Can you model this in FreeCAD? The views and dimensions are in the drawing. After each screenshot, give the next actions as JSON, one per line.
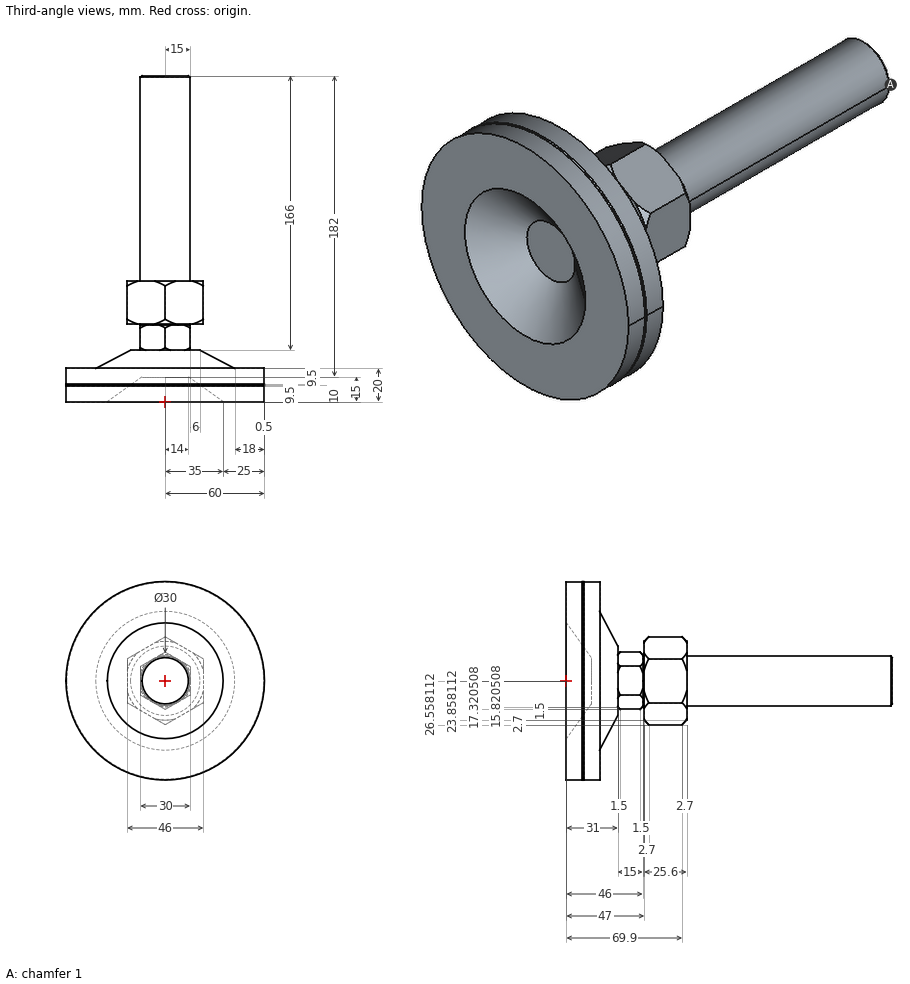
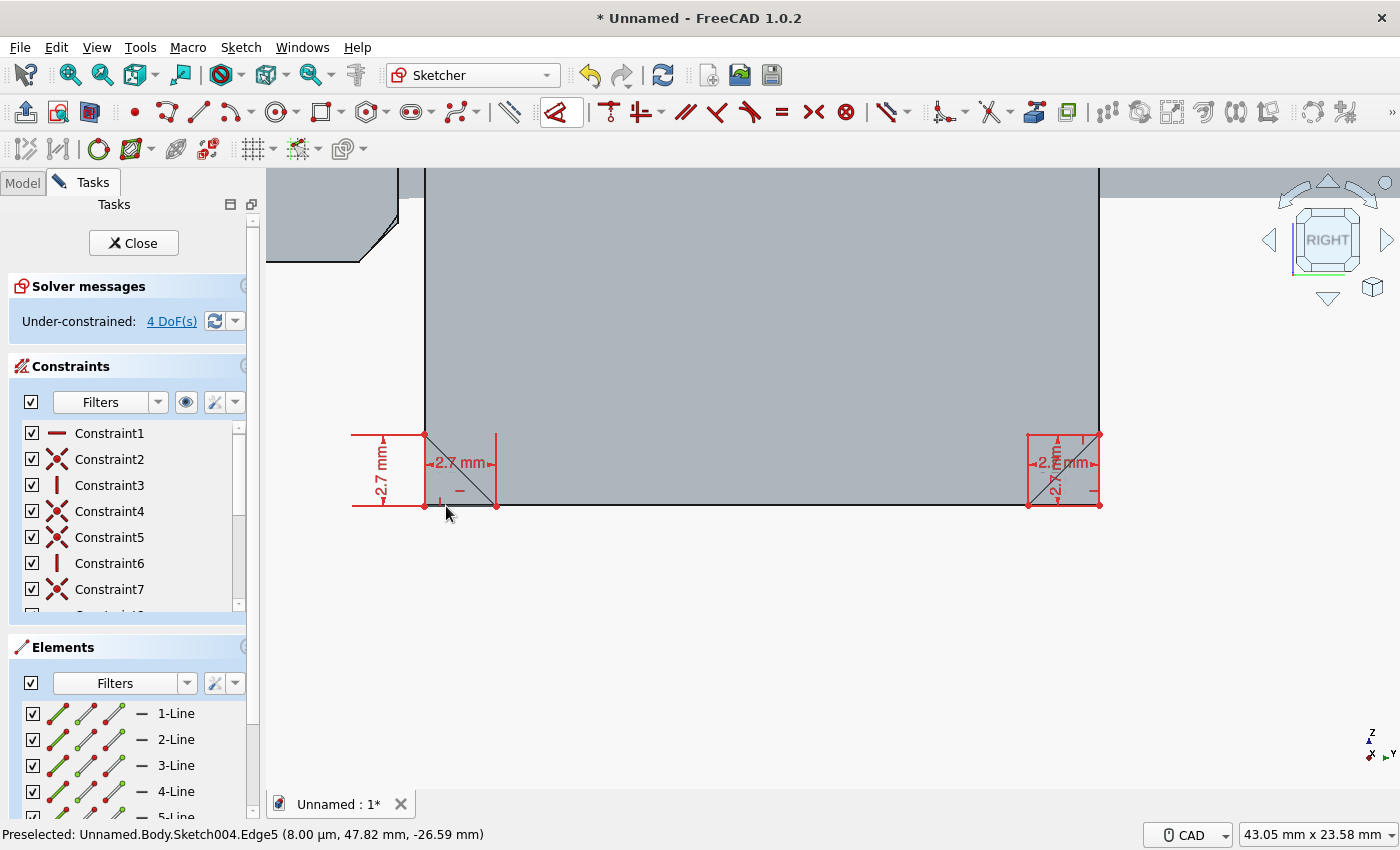
{"action": "left_click", "coordinate": [425, 435]}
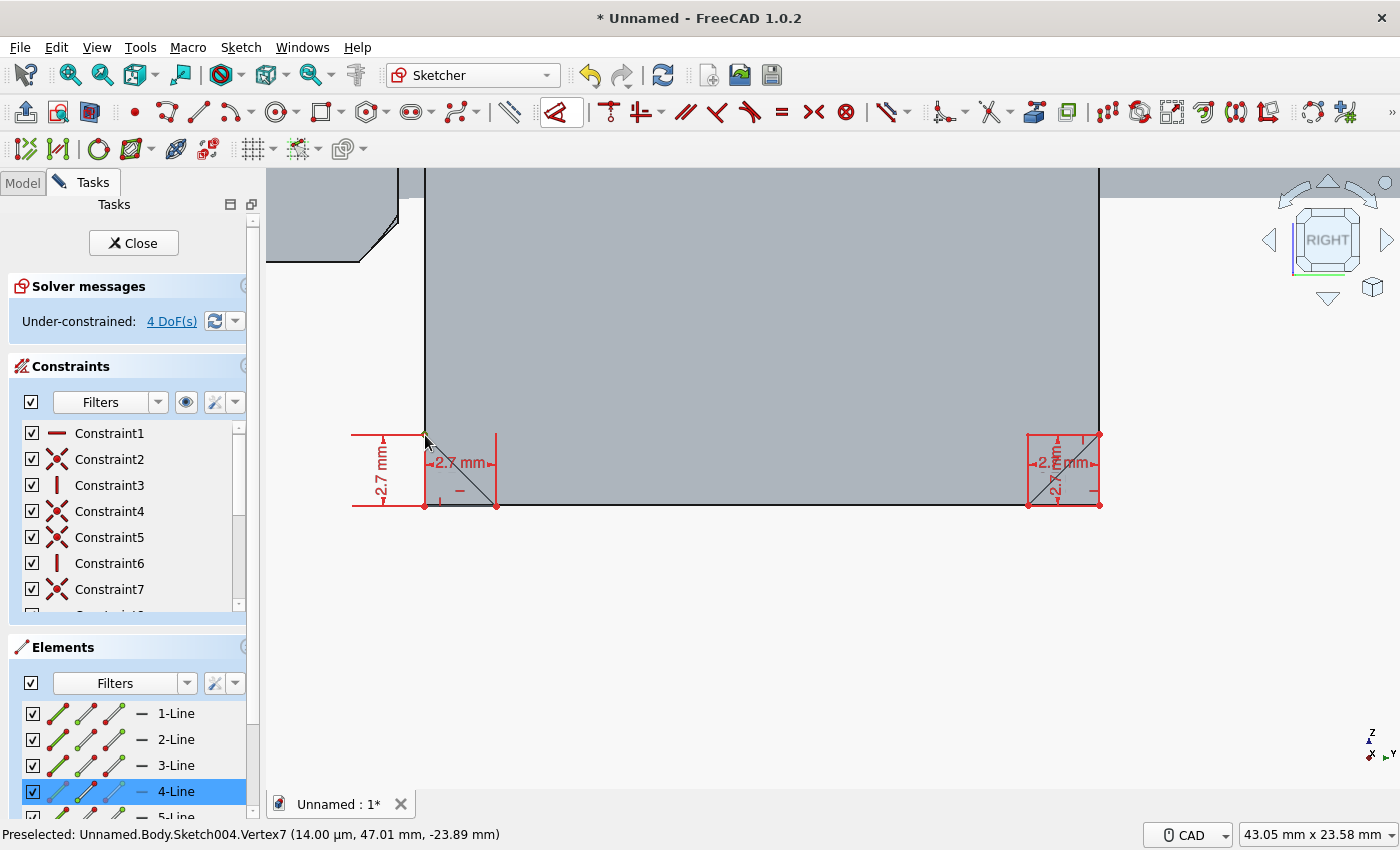
{"action": "key", "text": "l"}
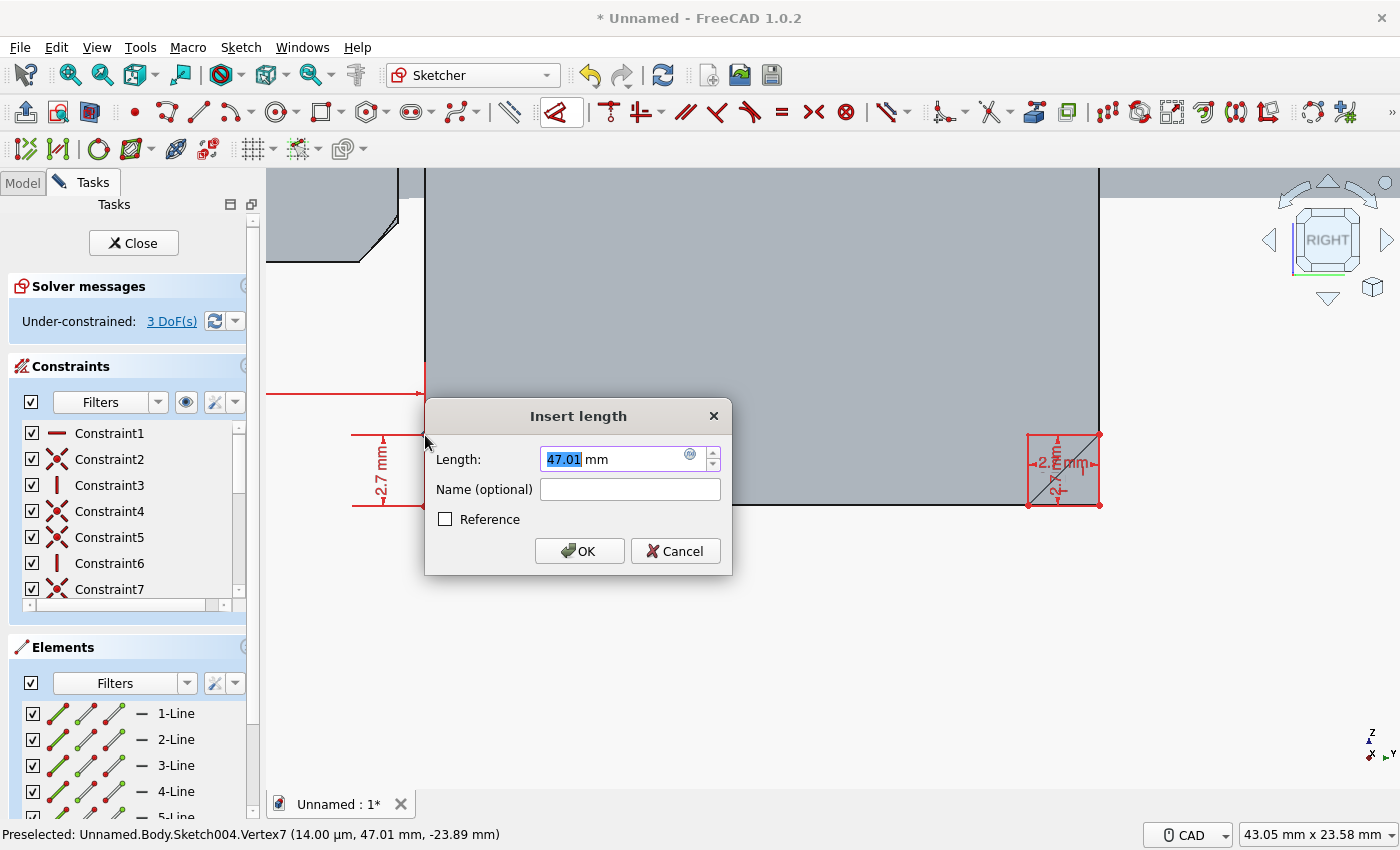
{"action": "type", "text": "47"}
{"action": "key", "text": "Return"}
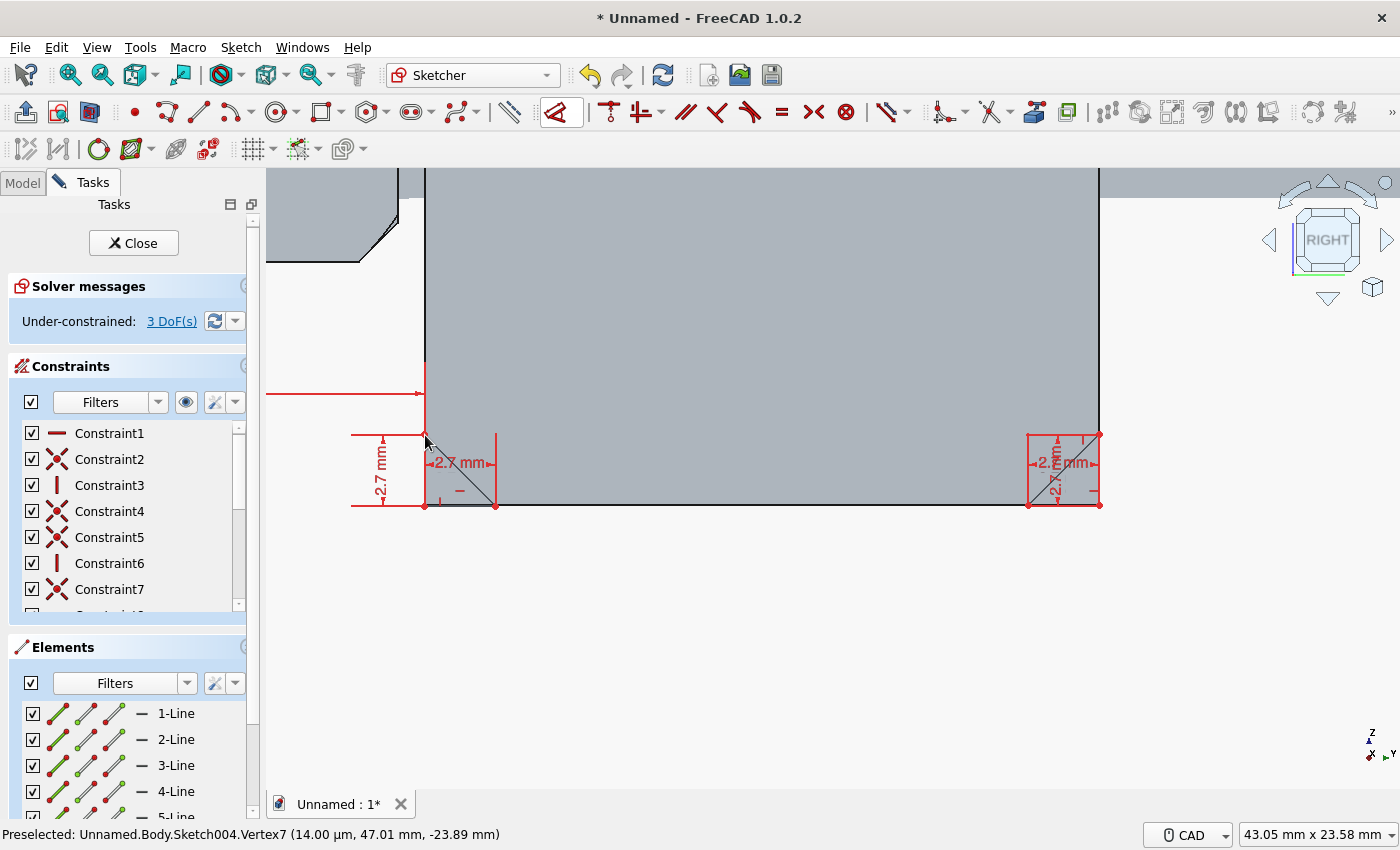
{"action": "left_click", "coordinate": [1028, 506]}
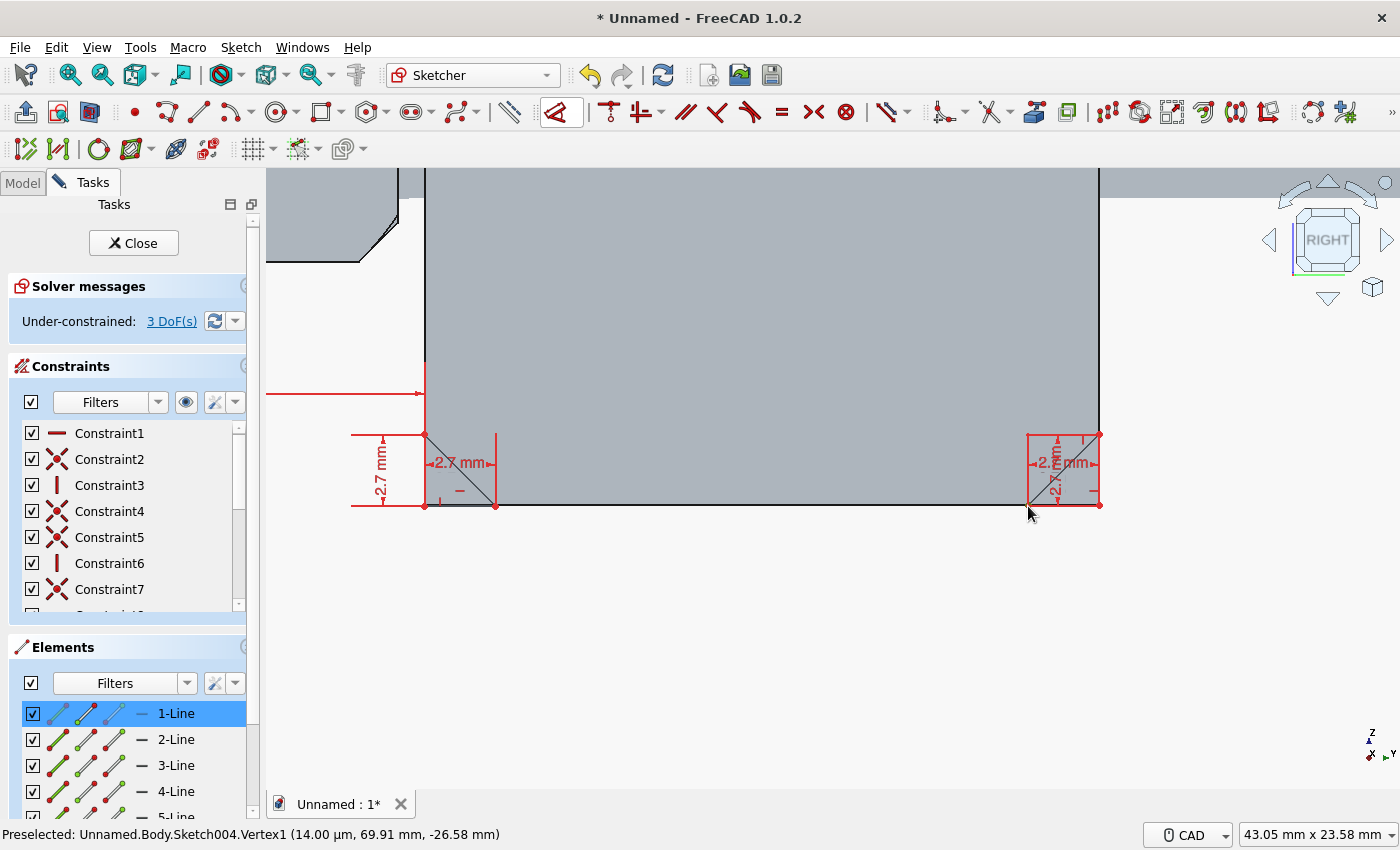
{"action": "left_click", "coordinate": [578, 112]}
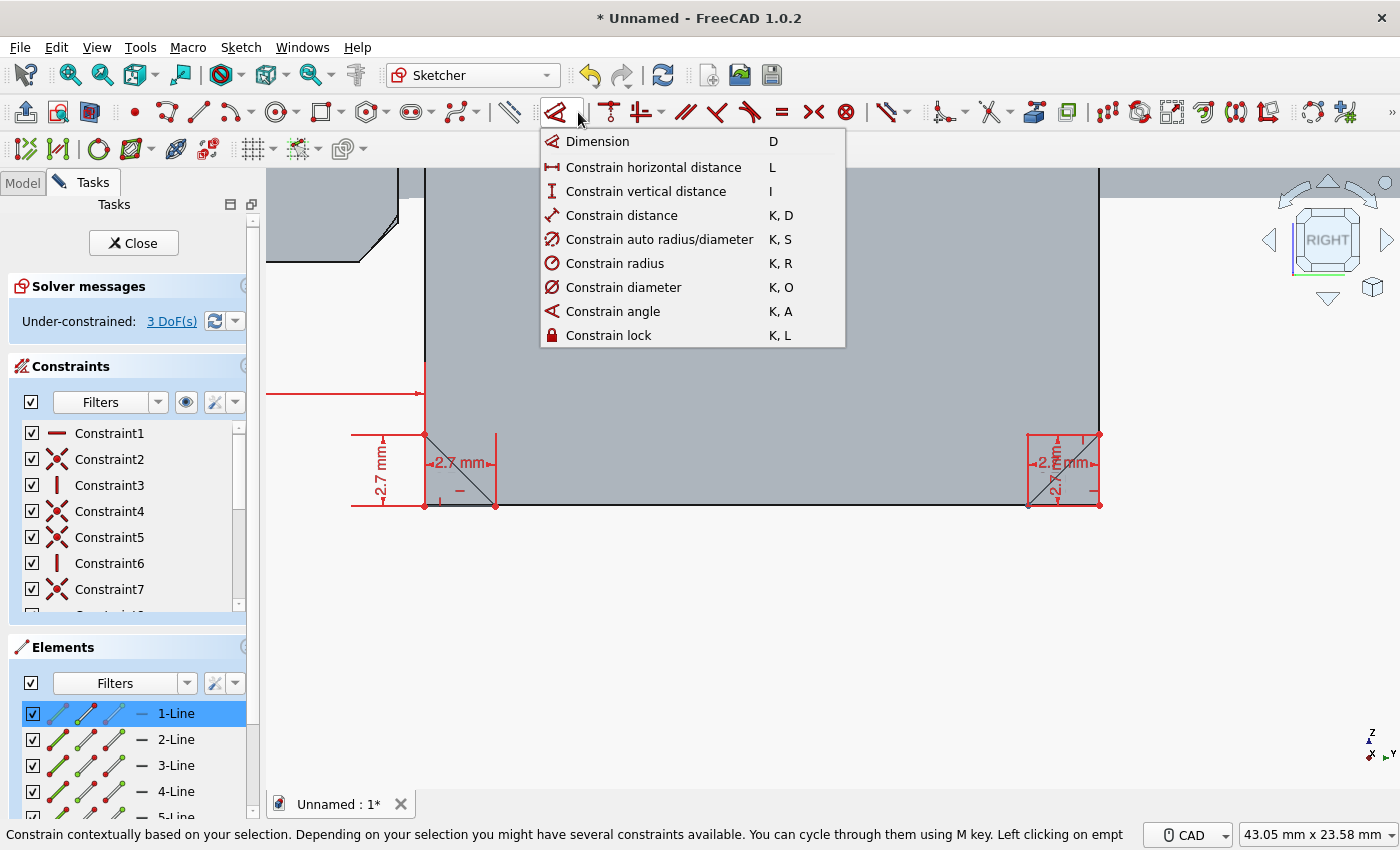
{"action": "left_click", "coordinate": [693, 167]}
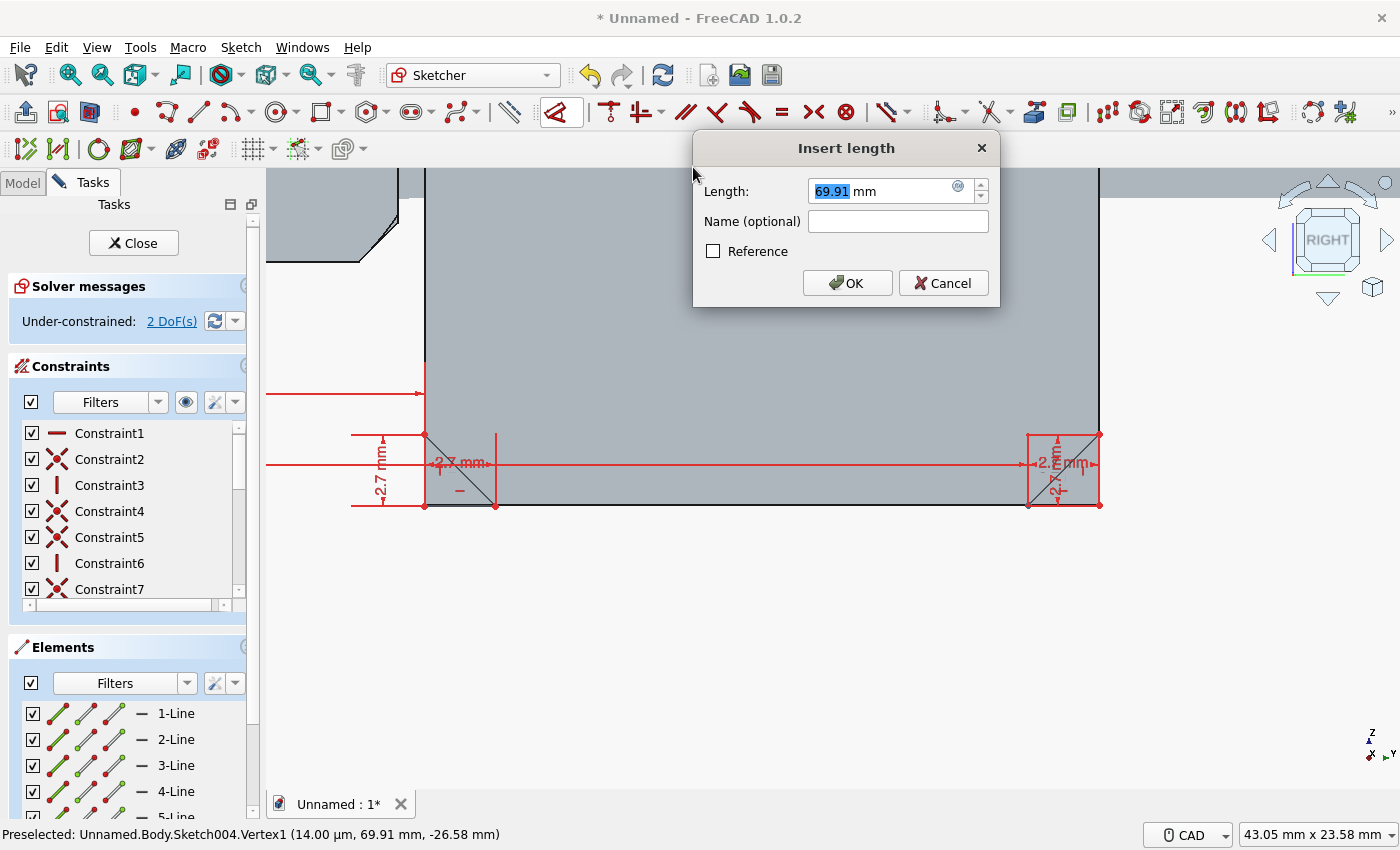
{"action": "type", "text": "69.9"}
{"action": "key", "text": "Return"}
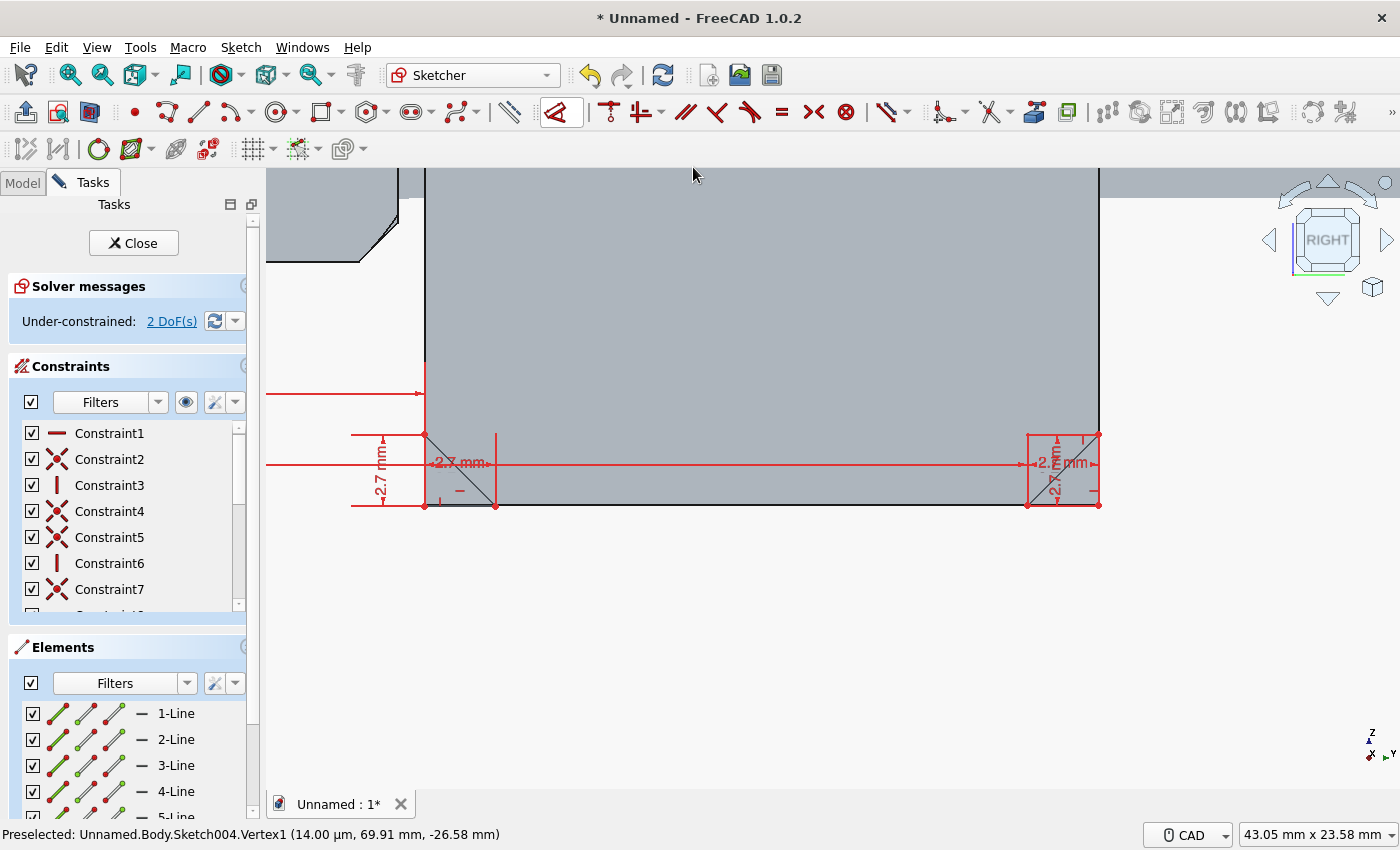
{"action": "left_click", "coordinate": [1028, 506]}